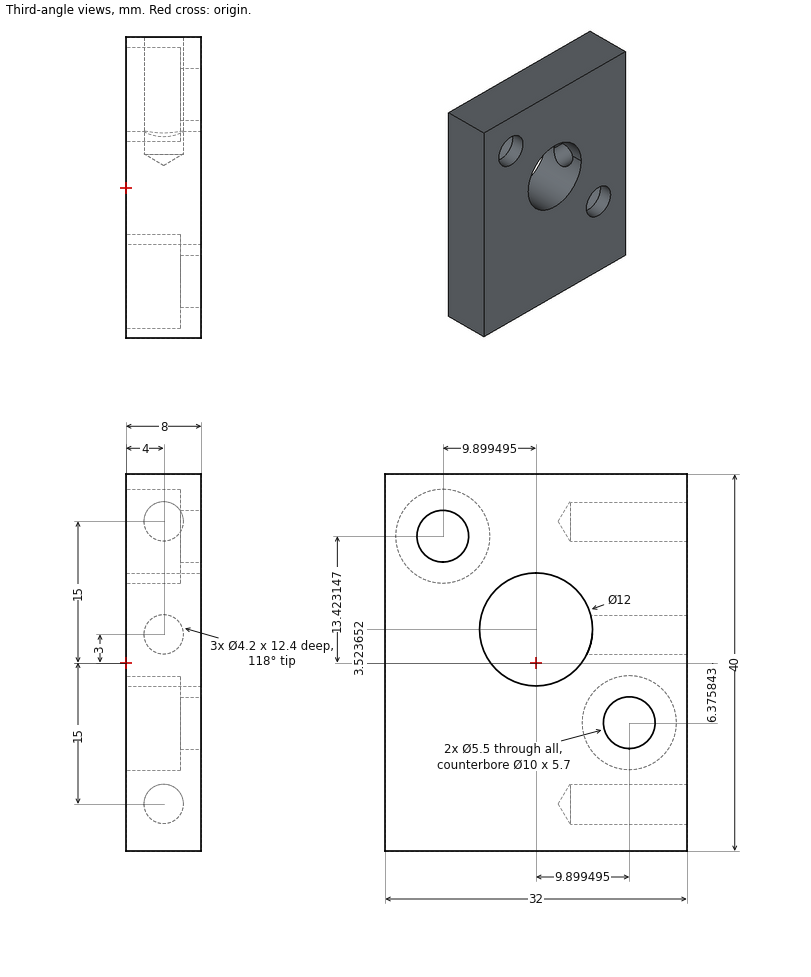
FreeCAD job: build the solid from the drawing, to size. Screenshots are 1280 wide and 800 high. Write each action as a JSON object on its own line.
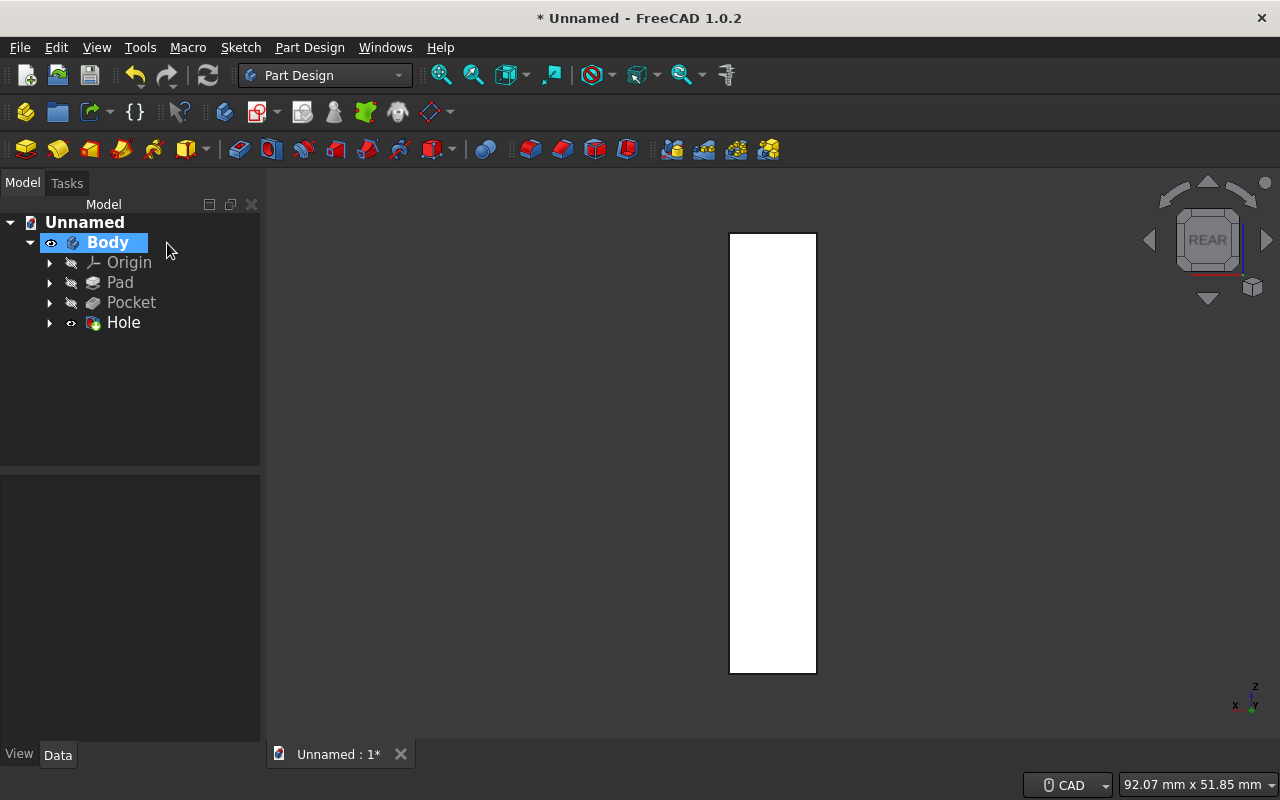
{"action": "left_click", "coordinate": [773, 453]}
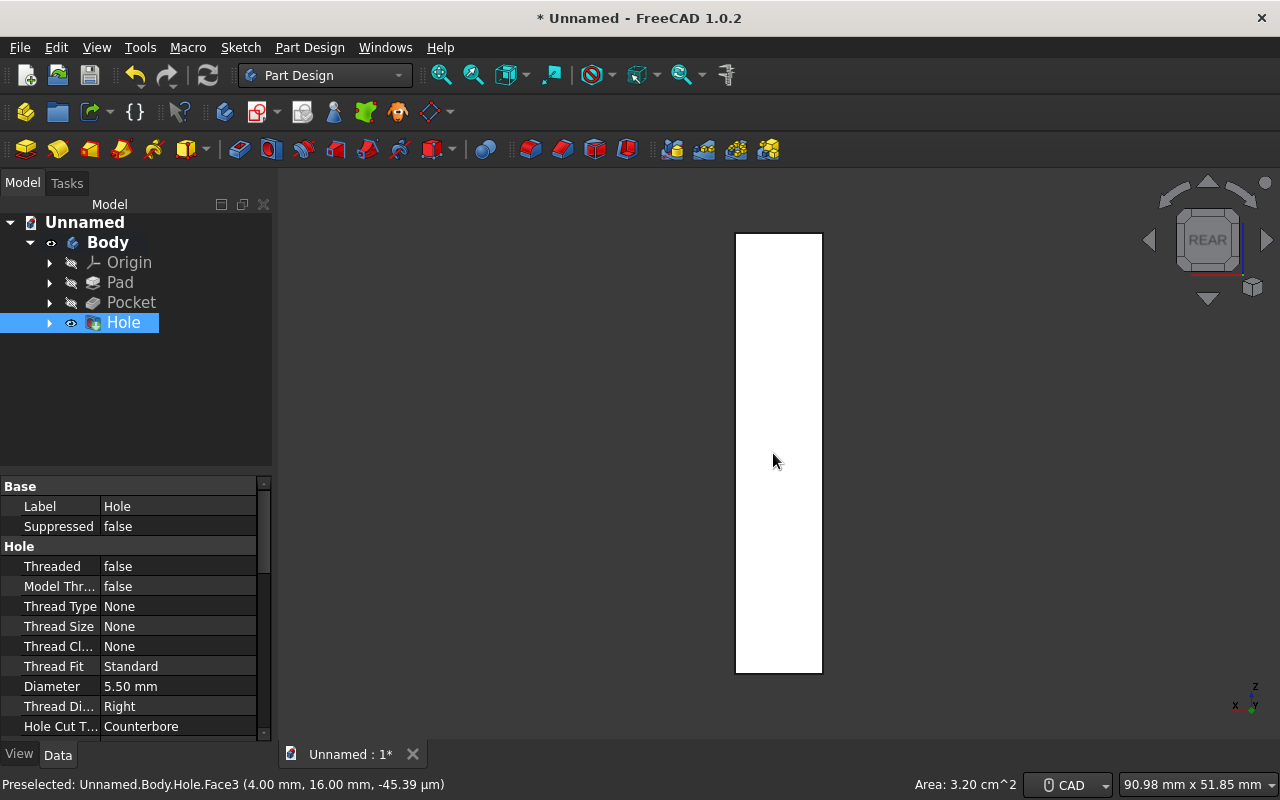
{"action": "left_click", "coordinate": [258, 112]}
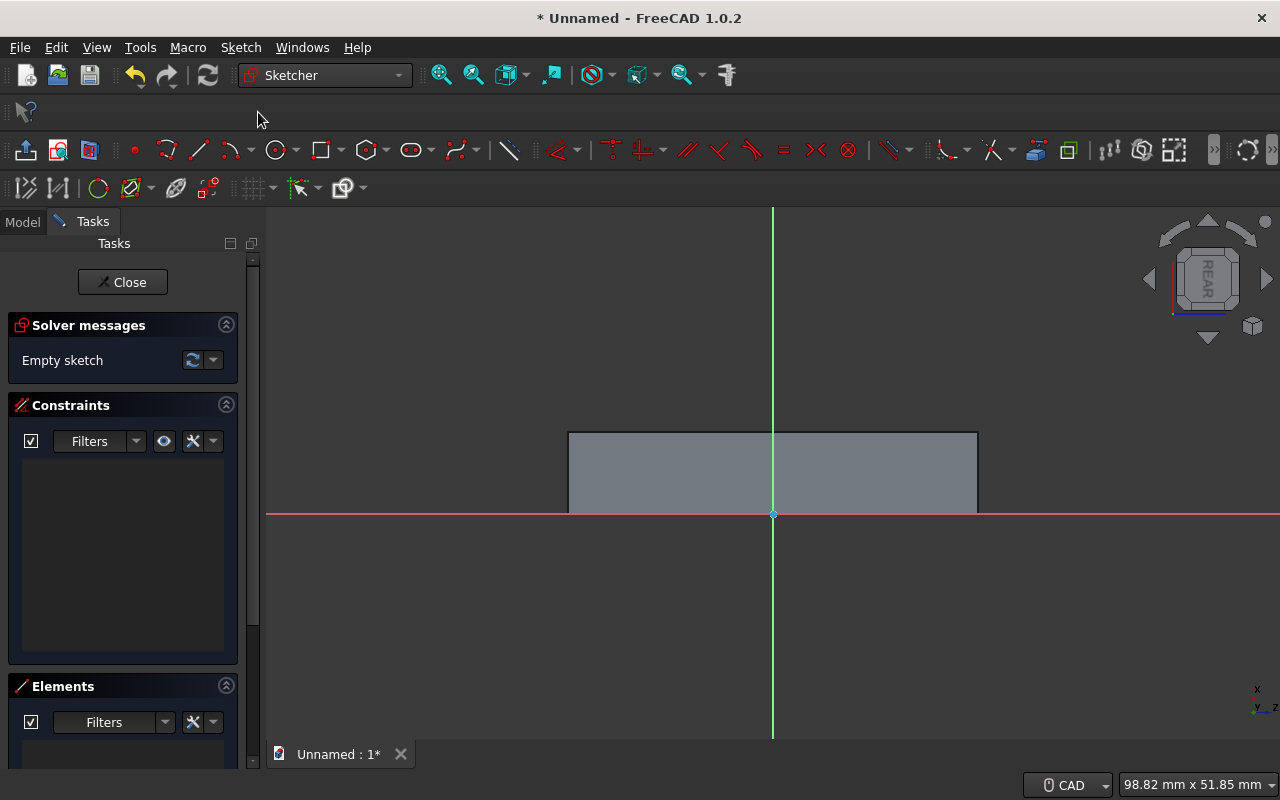
{"action": "scroll", "coordinate": [856, 495], "scroll_direction": "up", "scroll_amount": 3}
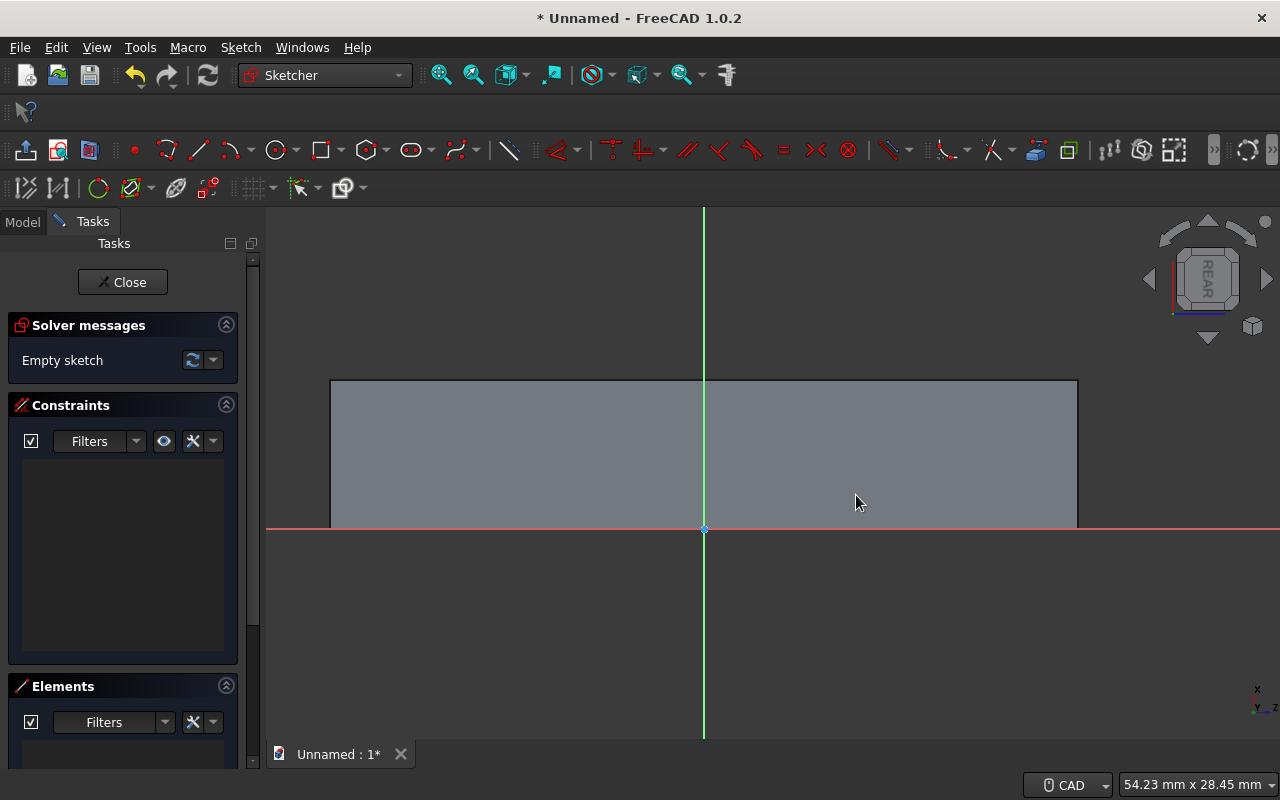
{"action": "key", "text": "g c"}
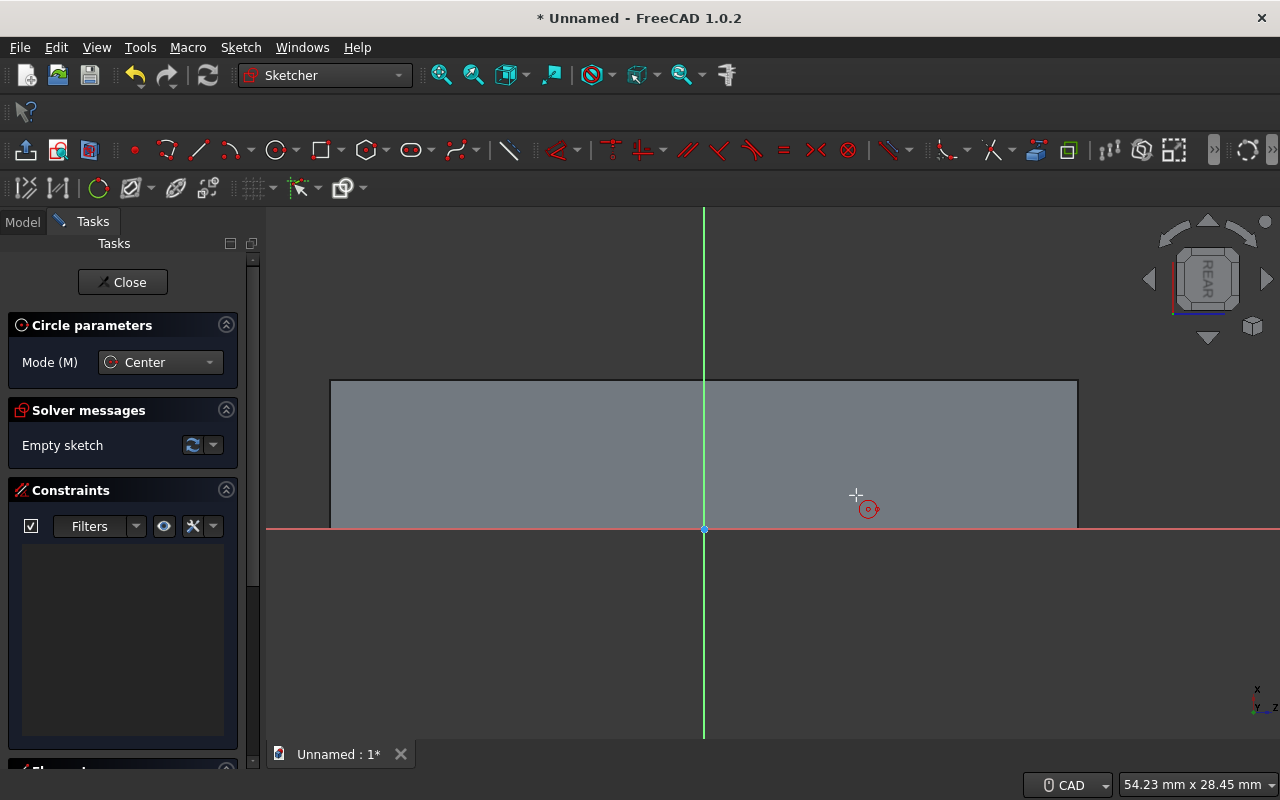
{"action": "left_click", "coordinate": [760, 454]}
{"action": "mouse_move", "coordinate": [788, 427]}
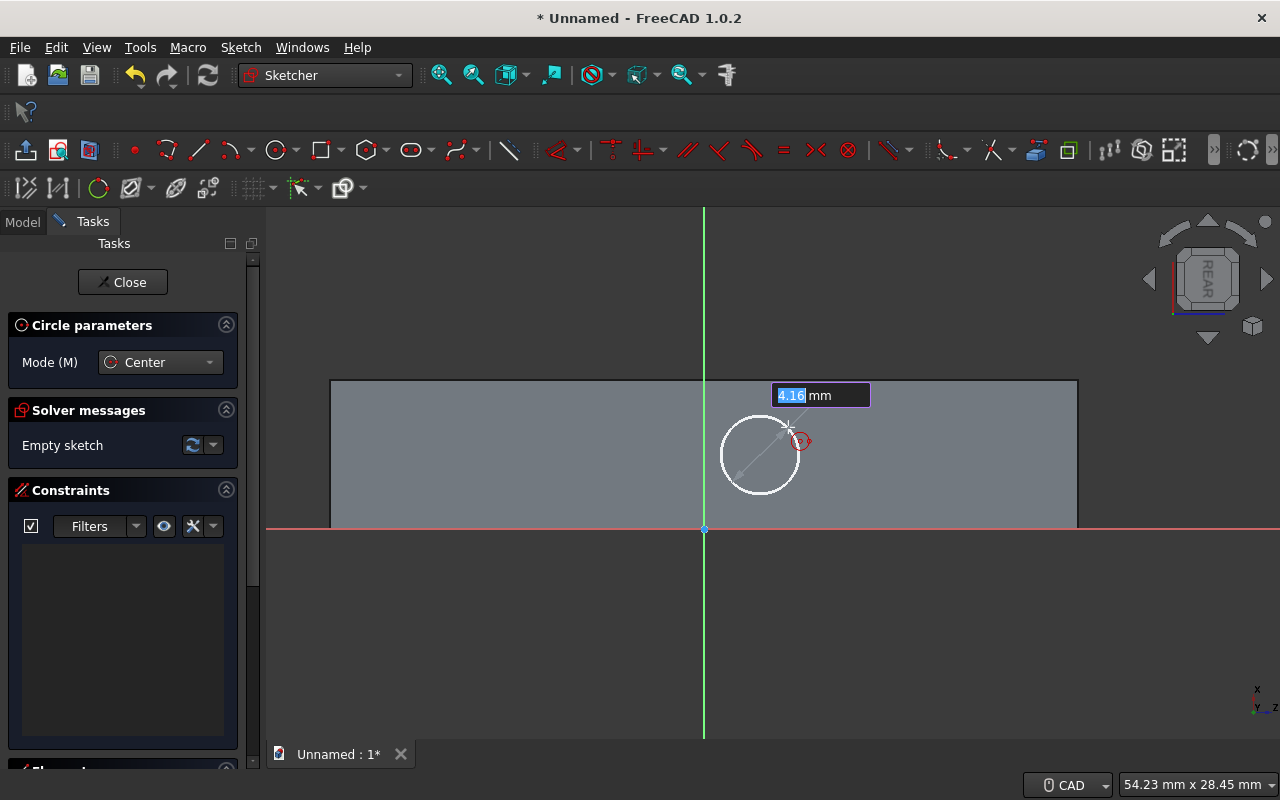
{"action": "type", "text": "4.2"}
{"action": "key", "text": "Return"}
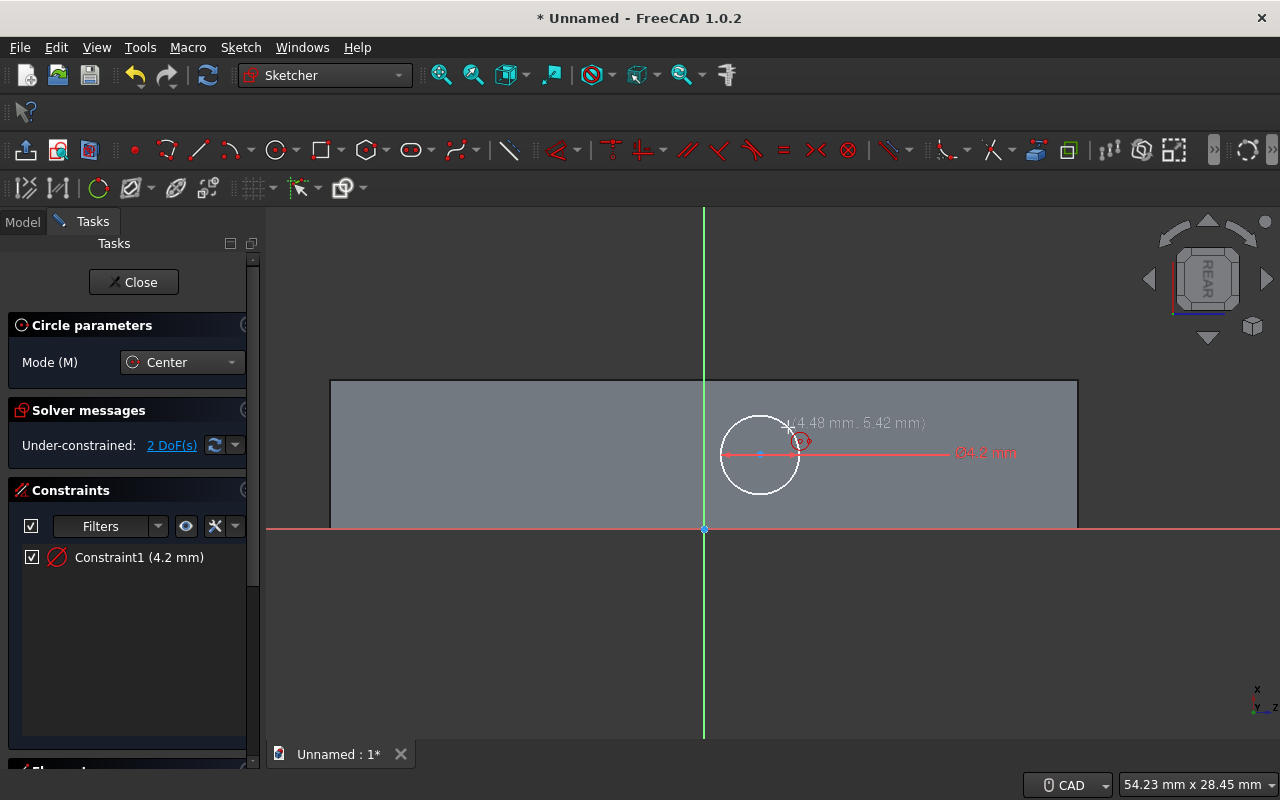
{"action": "left_click", "coordinate": [985, 454]}
{"action": "mouse_move", "coordinate": [1013, 427]}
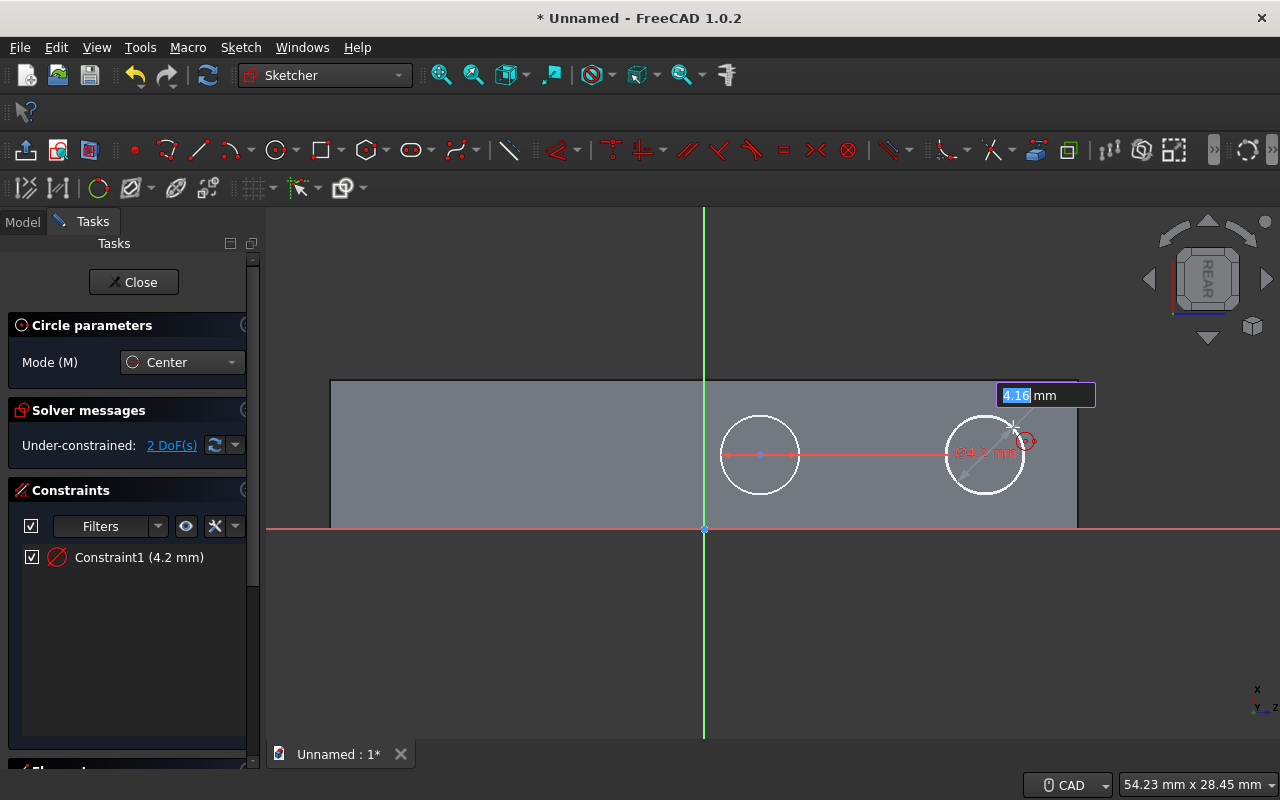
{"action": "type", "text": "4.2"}
{"action": "key", "text": "Return"}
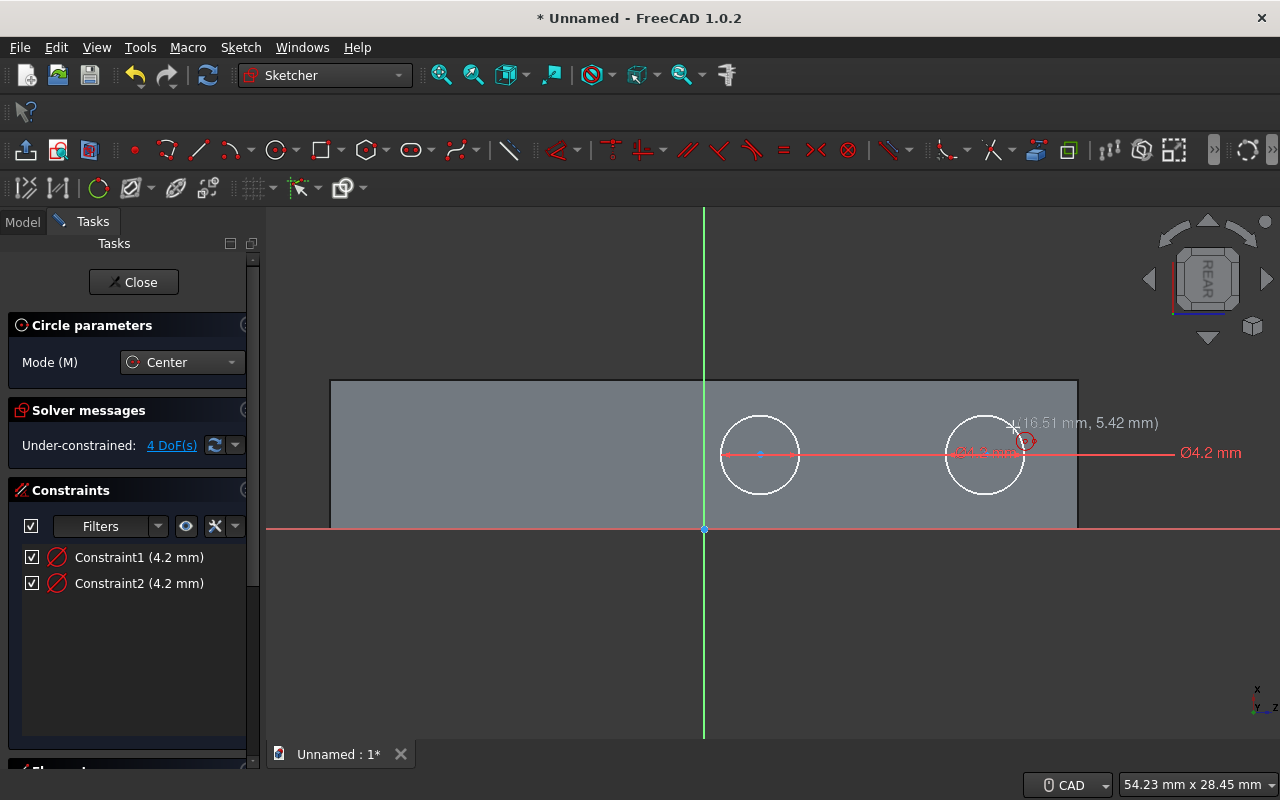
{"action": "left_click", "coordinate": [424, 454]}
{"action": "mouse_move", "coordinate": [452, 427]}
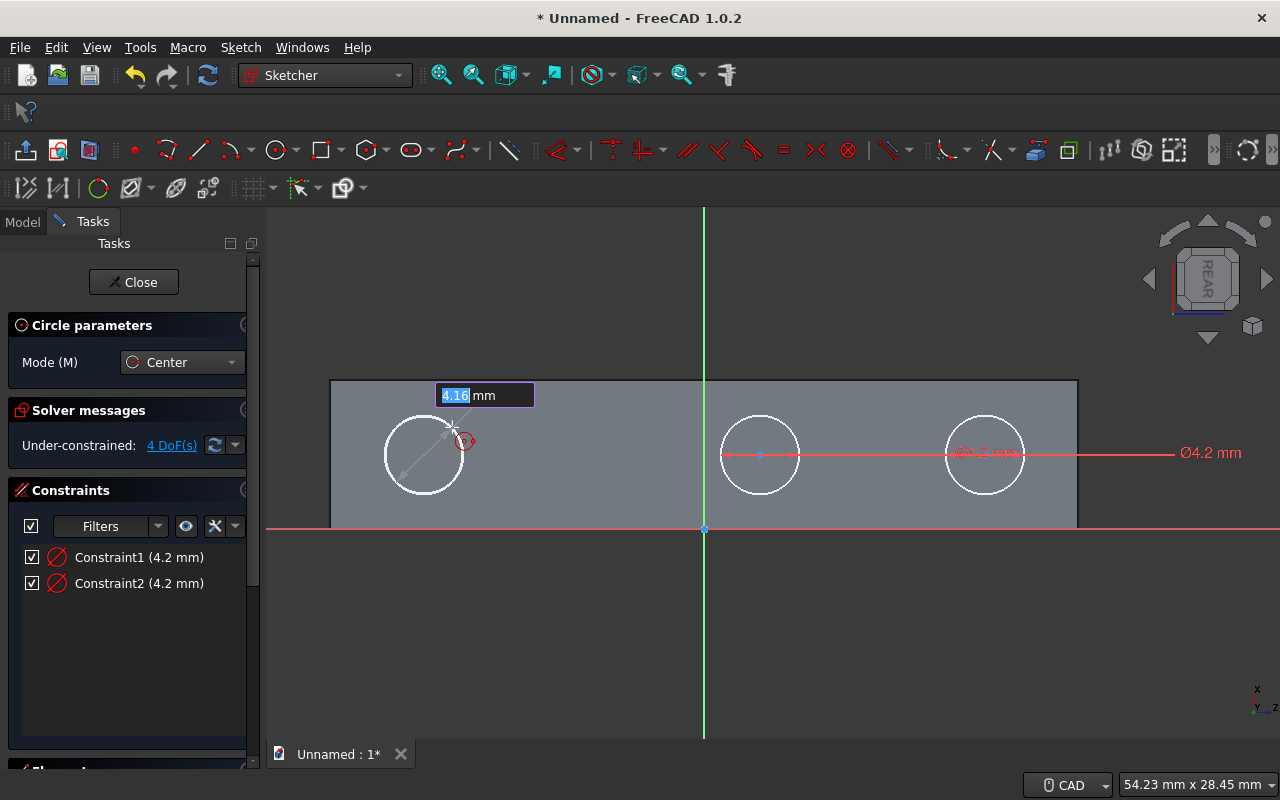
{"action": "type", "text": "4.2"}
{"action": "key", "text": "Return"}
{"action": "key", "text": "Escape"}